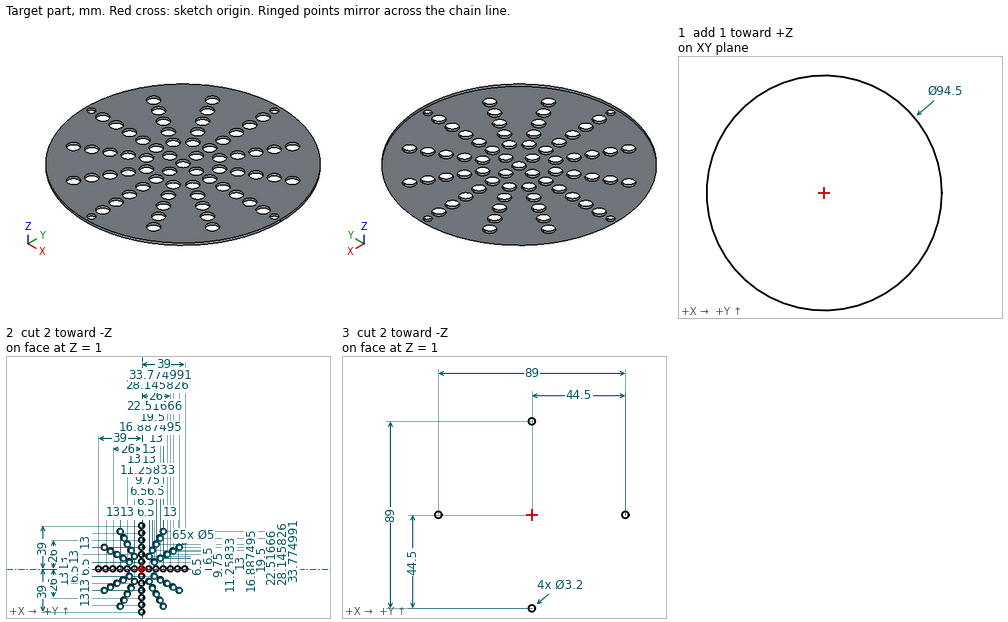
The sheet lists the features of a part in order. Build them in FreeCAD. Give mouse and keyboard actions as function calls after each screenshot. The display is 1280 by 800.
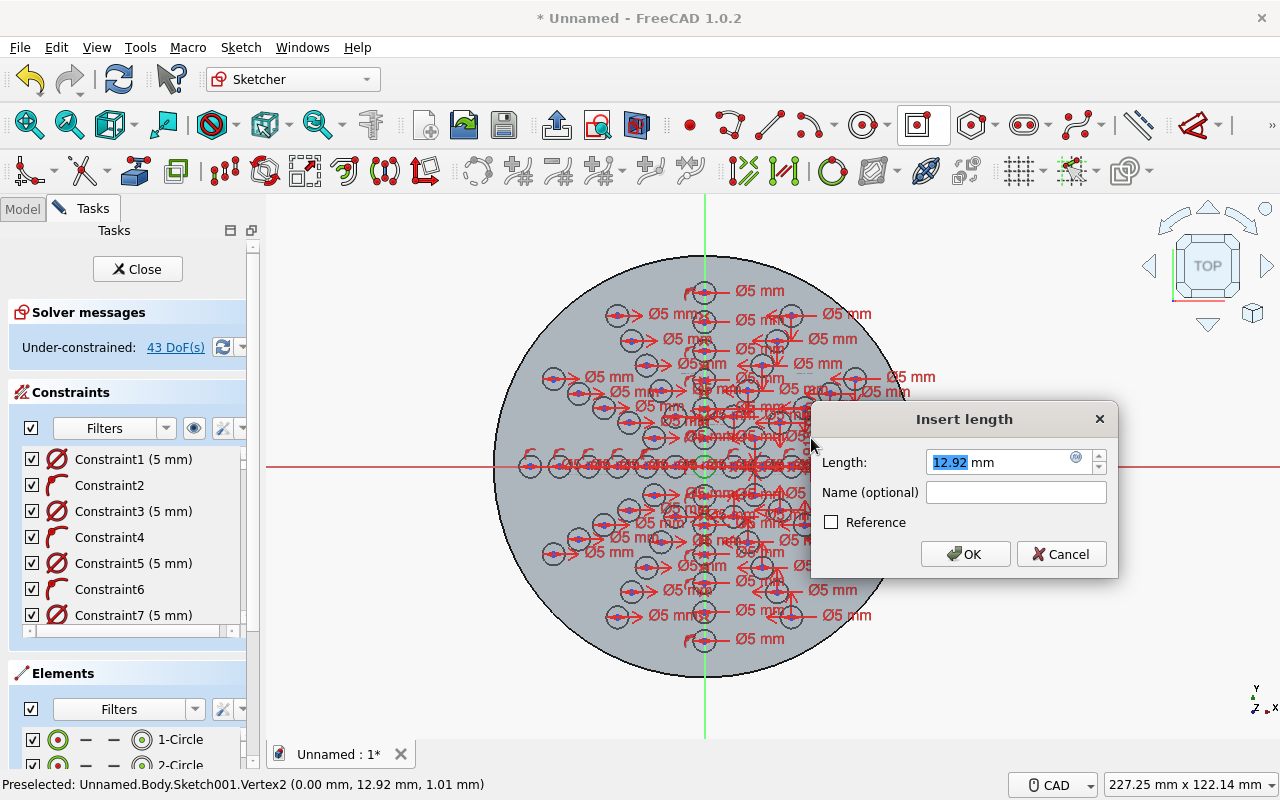
text(13)
key(Return)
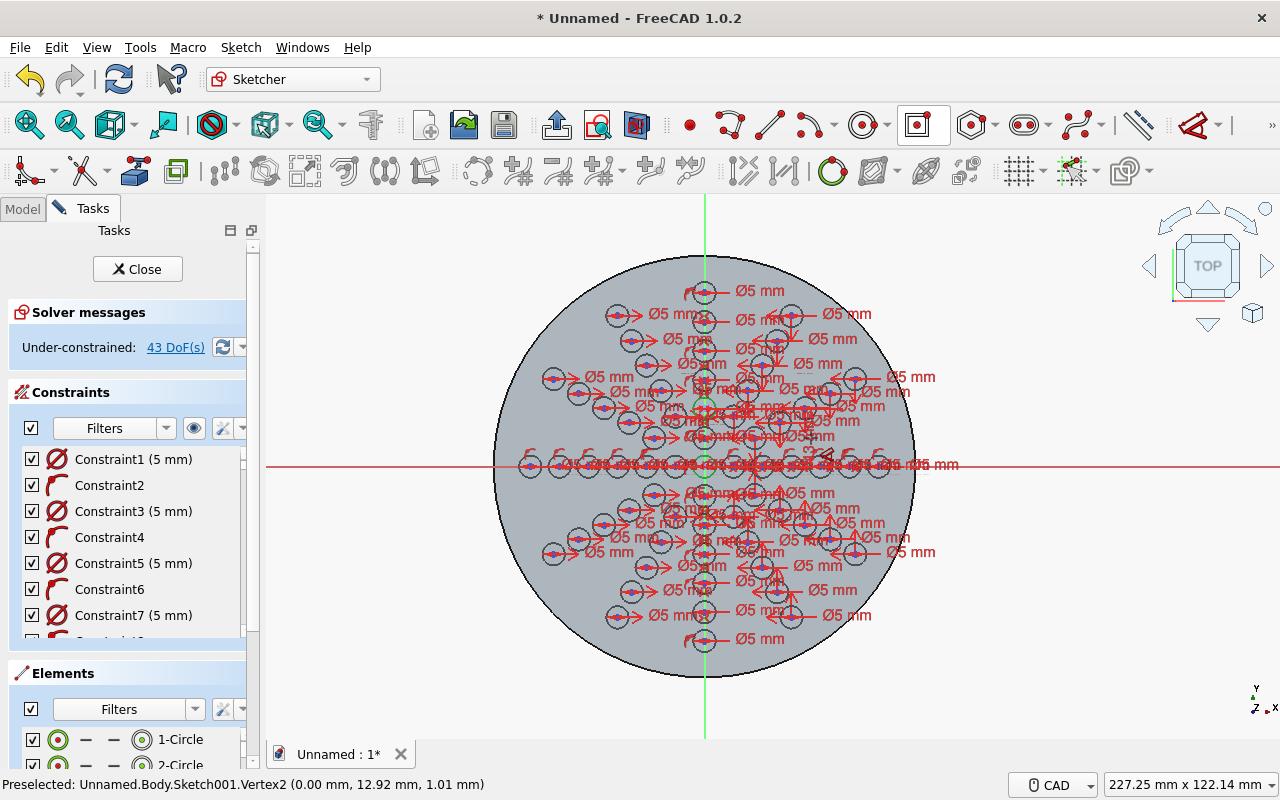
click(705, 351)
click(787, 382)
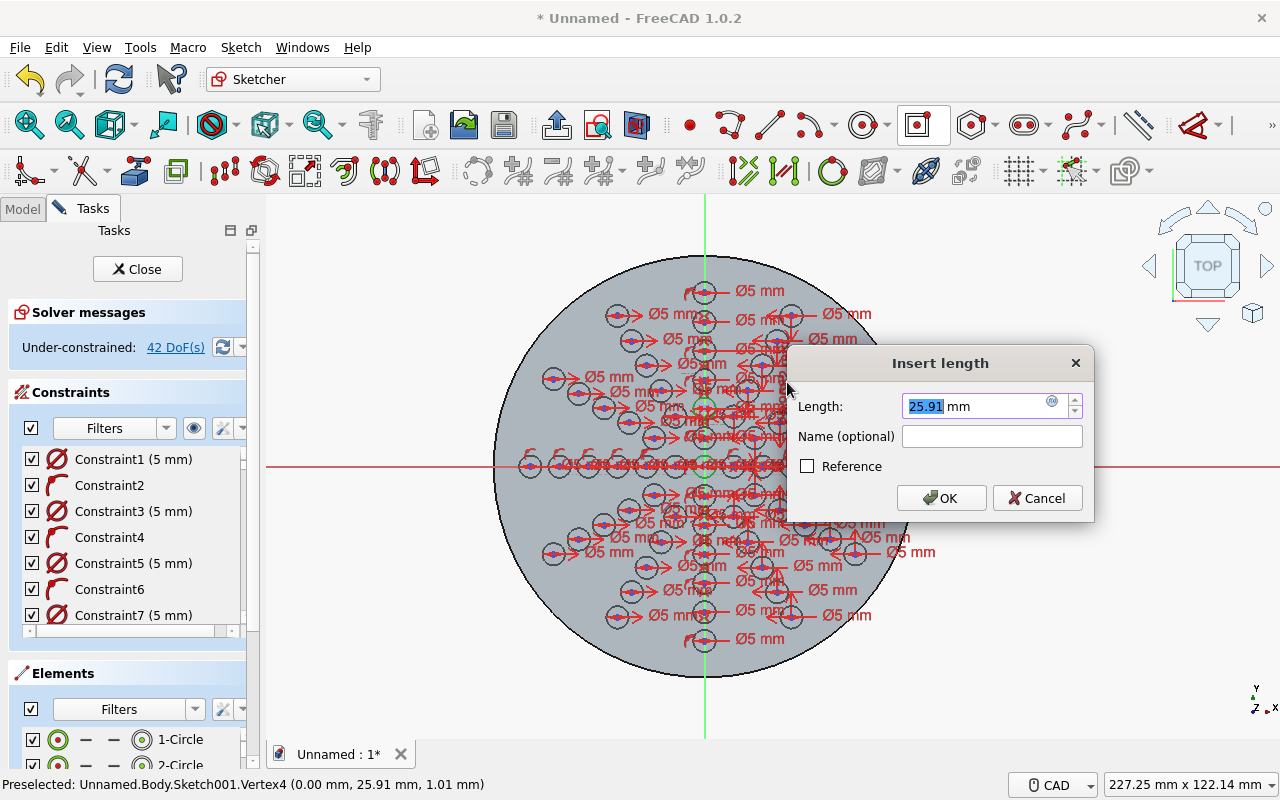
text(26)
key(Return)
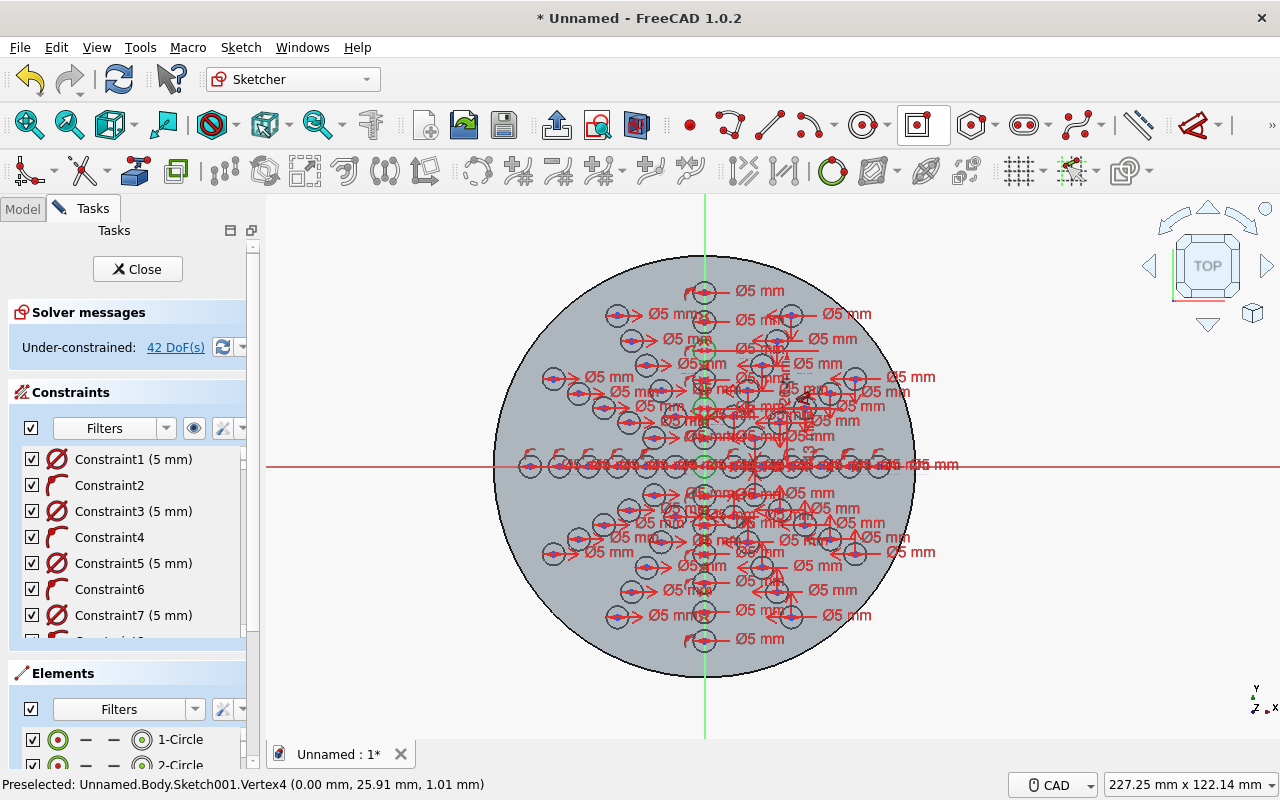
click(705, 293)
click(739, 340)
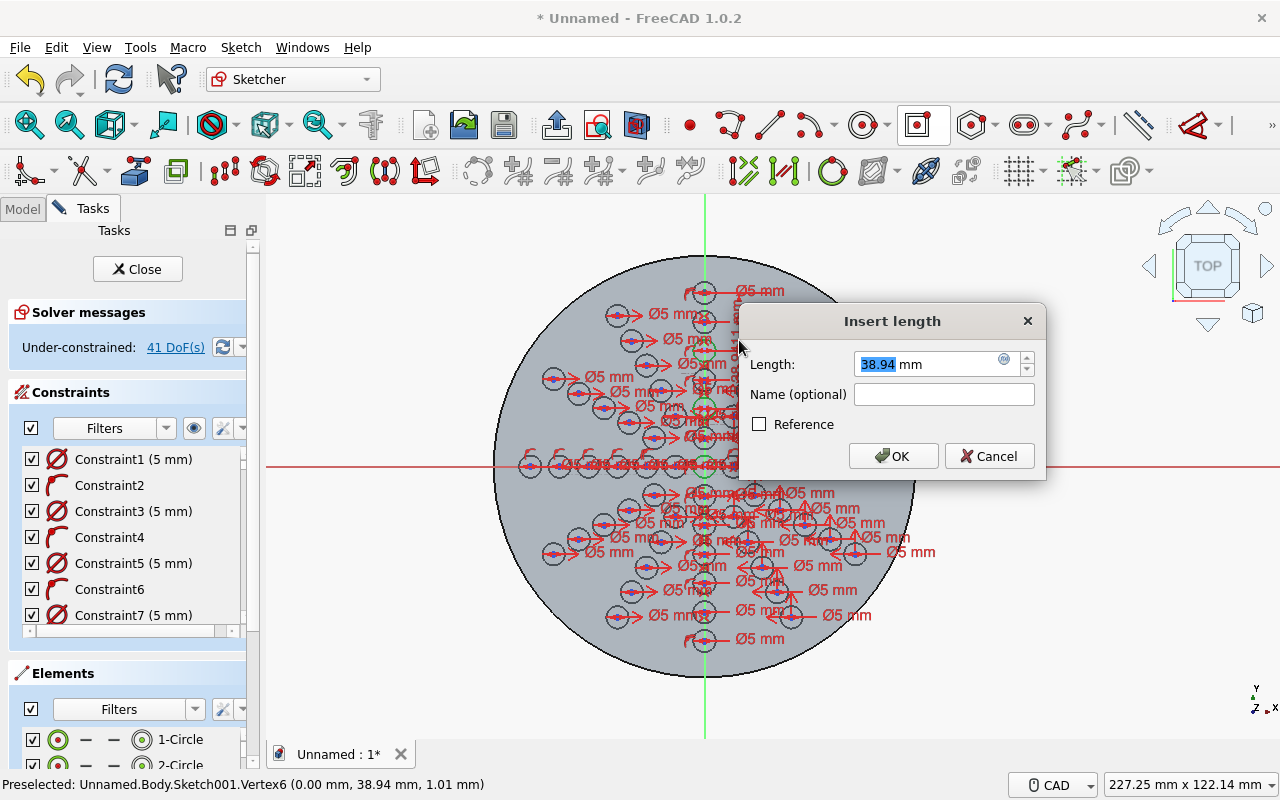
text(39)
key(Return)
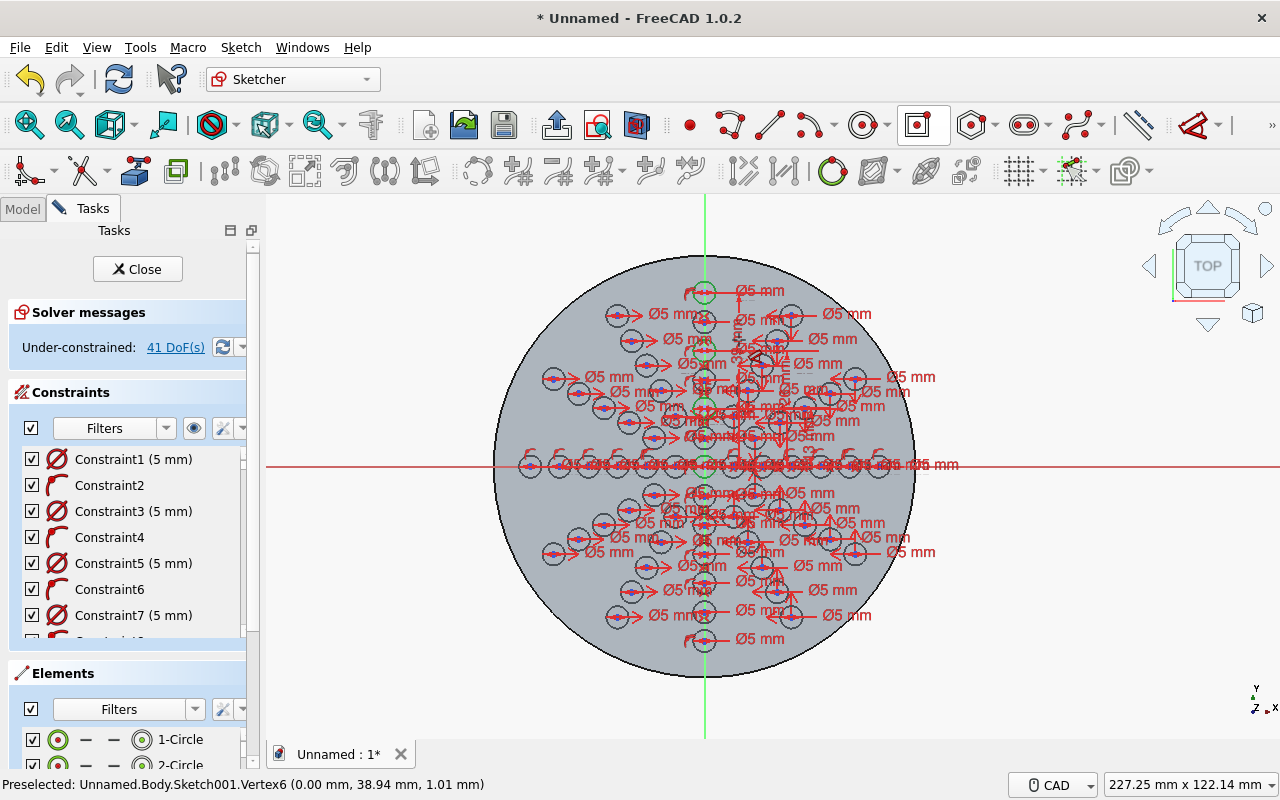
click(762, 366)
click(733, 308)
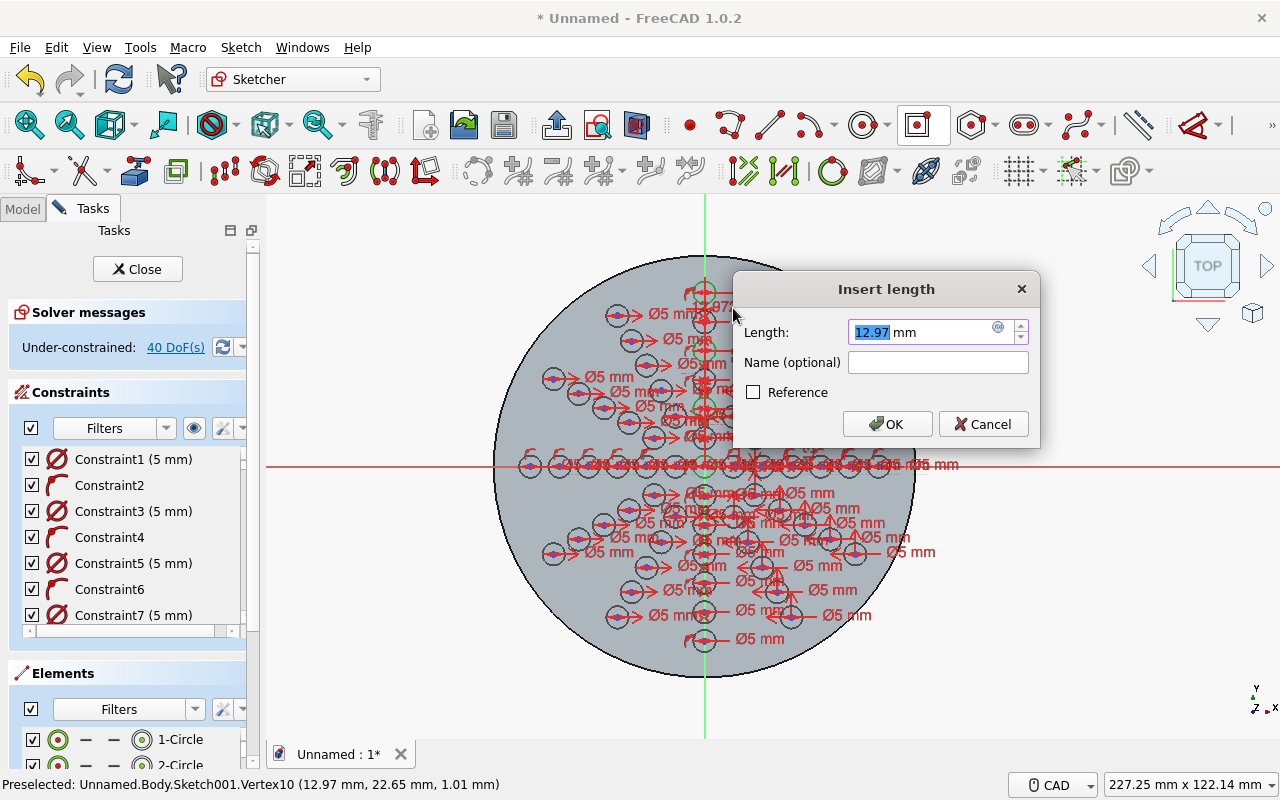
text(13)
key(Return)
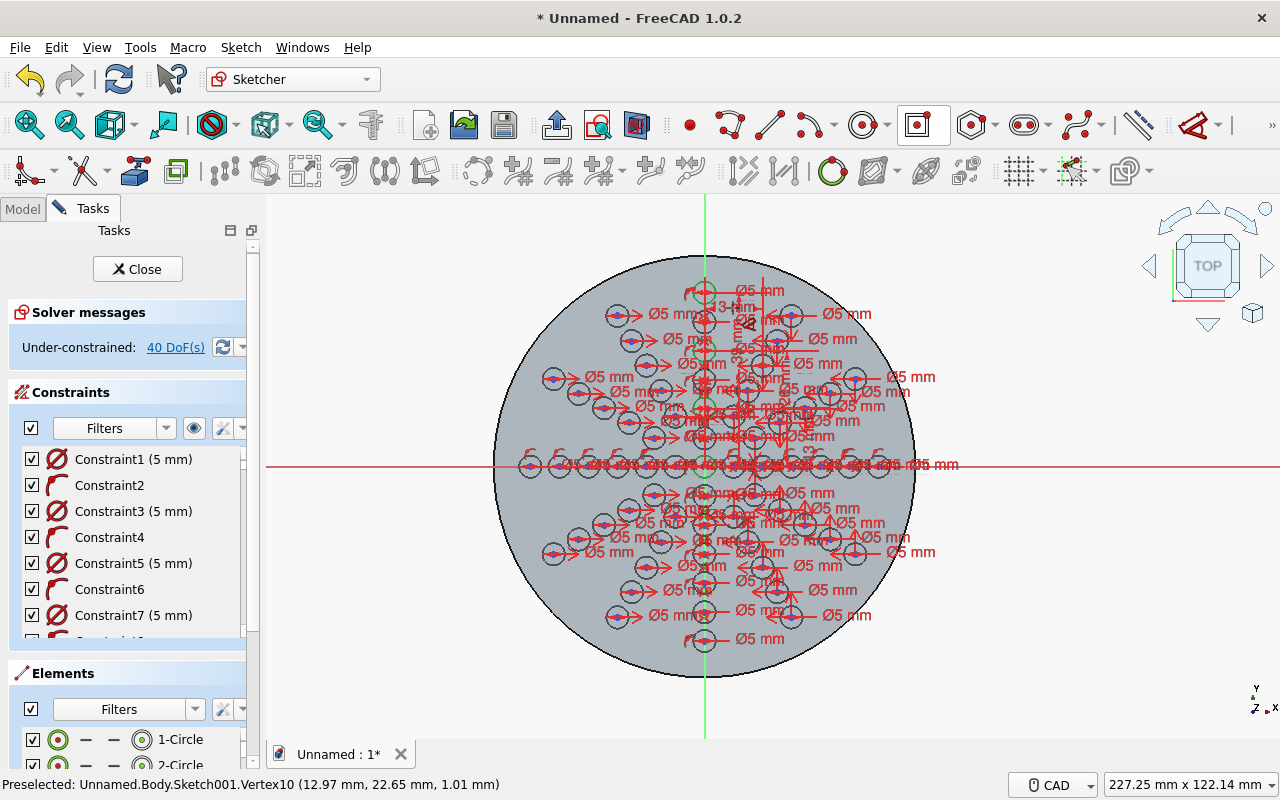
click(805, 408)
click(839, 417)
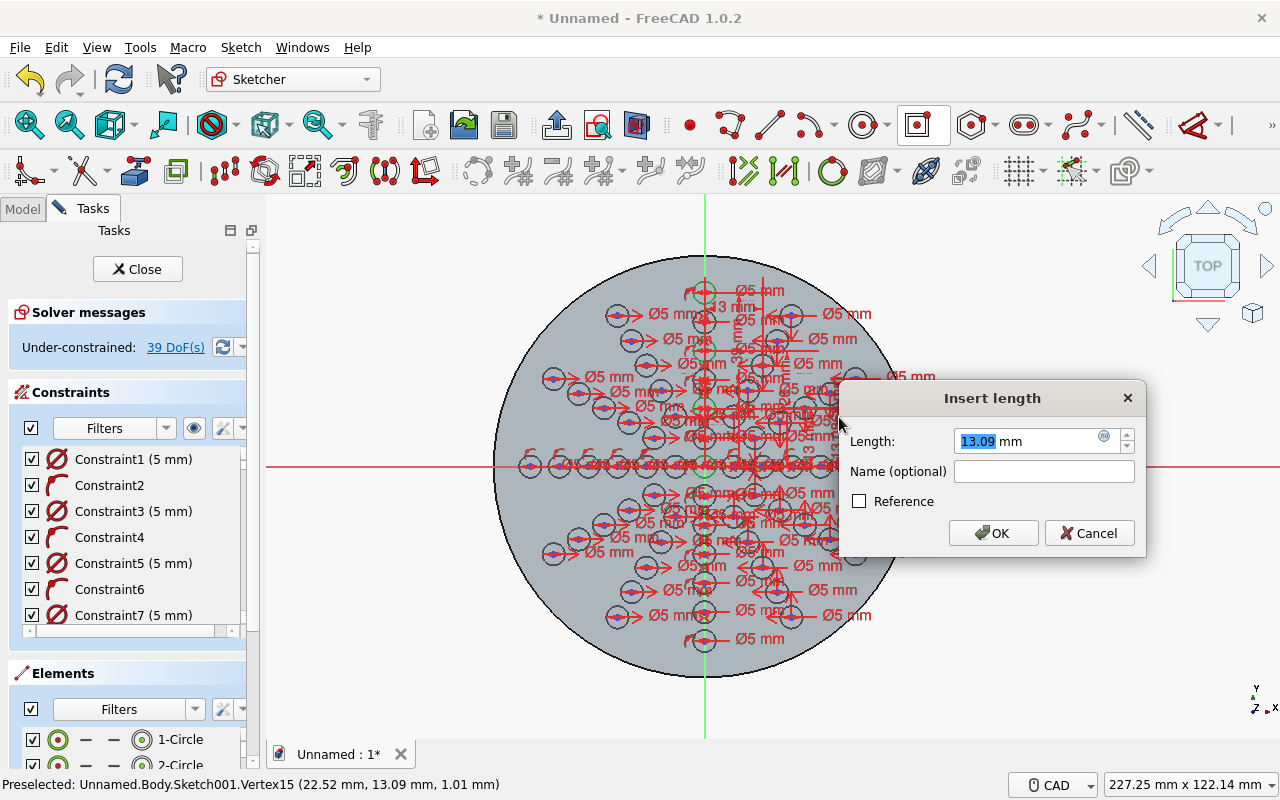
text(13)
key(Return)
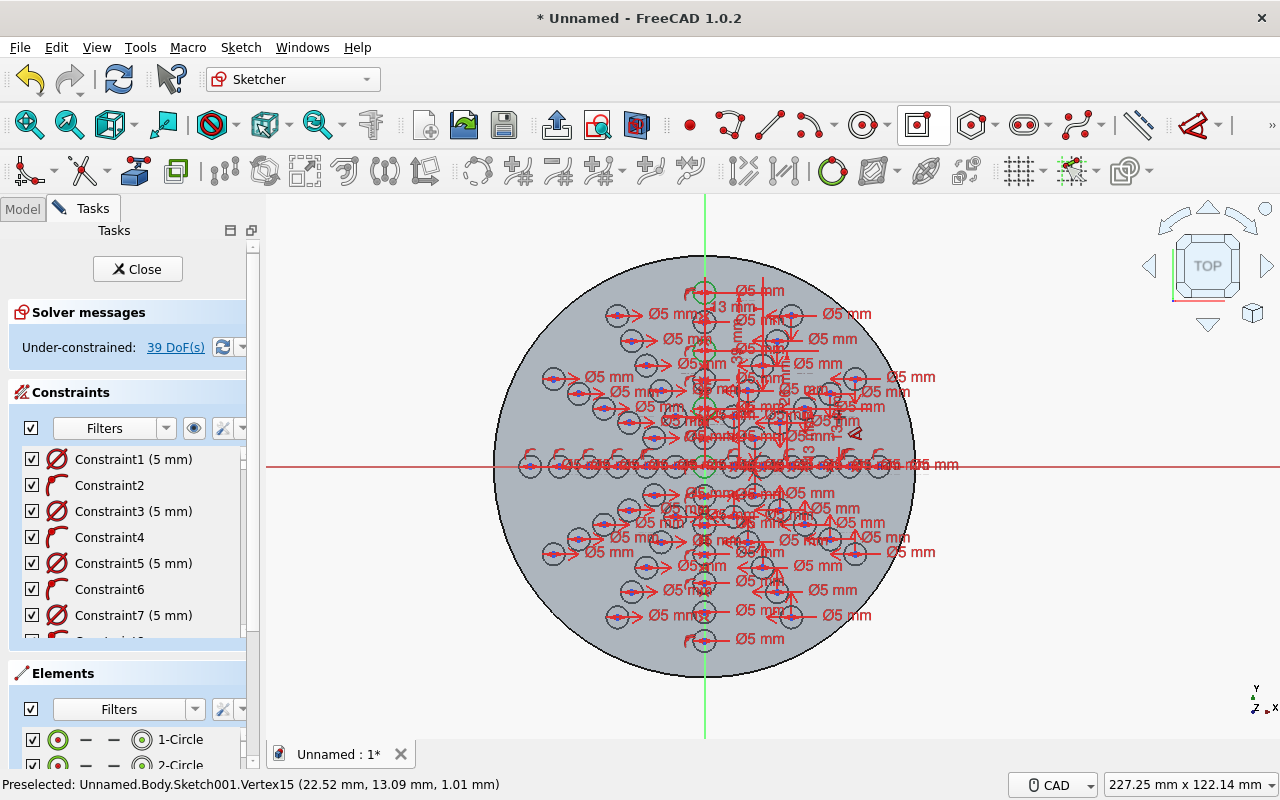
click(879, 467)
click(832, 501)